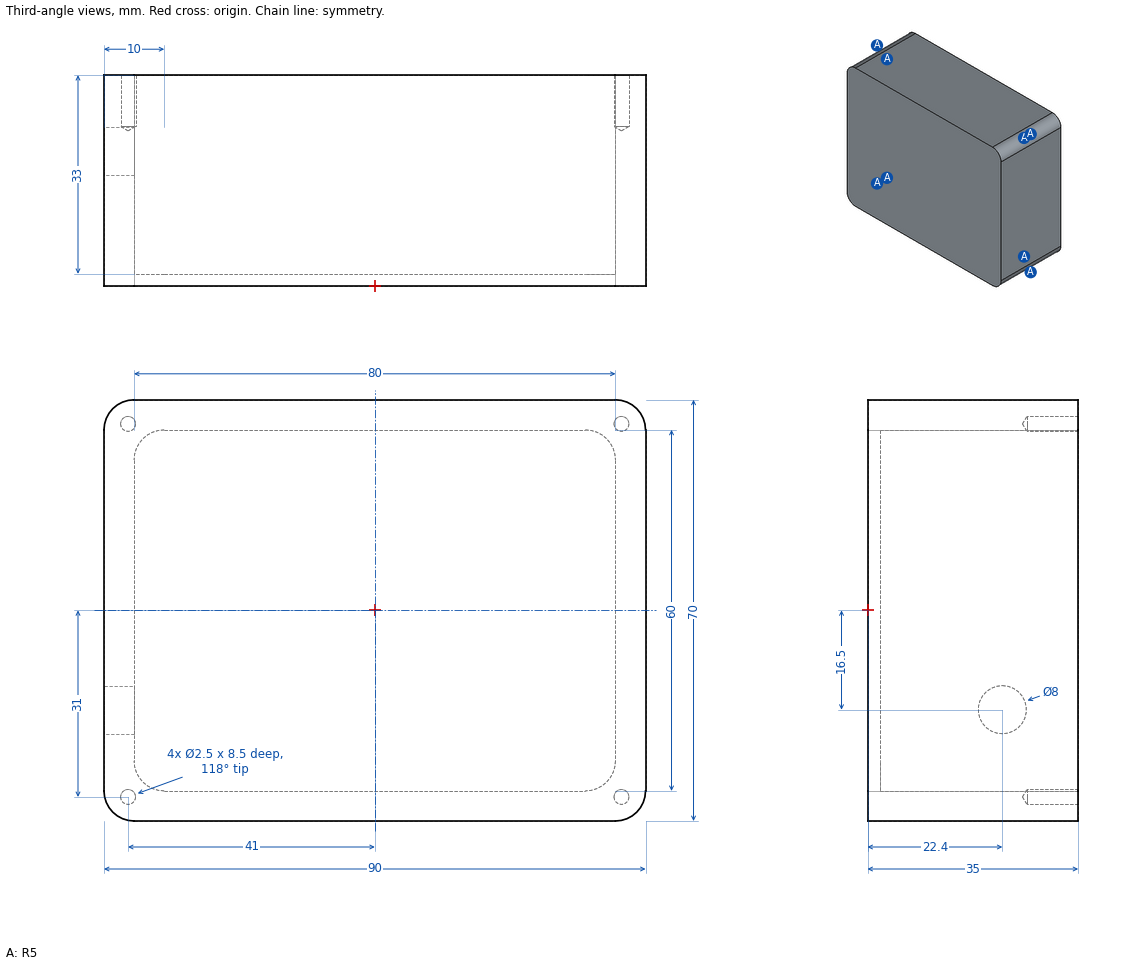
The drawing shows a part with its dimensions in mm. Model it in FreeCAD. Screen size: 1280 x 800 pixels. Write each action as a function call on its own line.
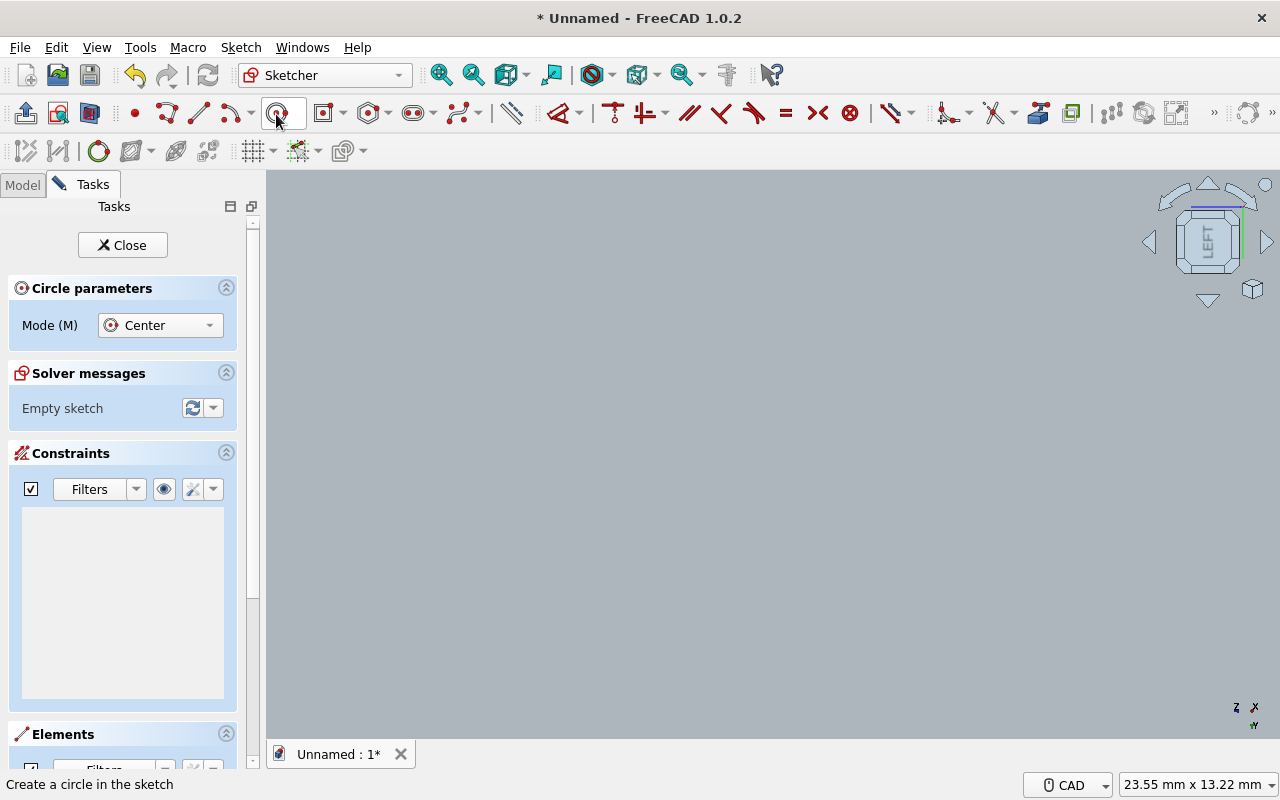
click(700, 448)
click(822, 327)
key(Escape)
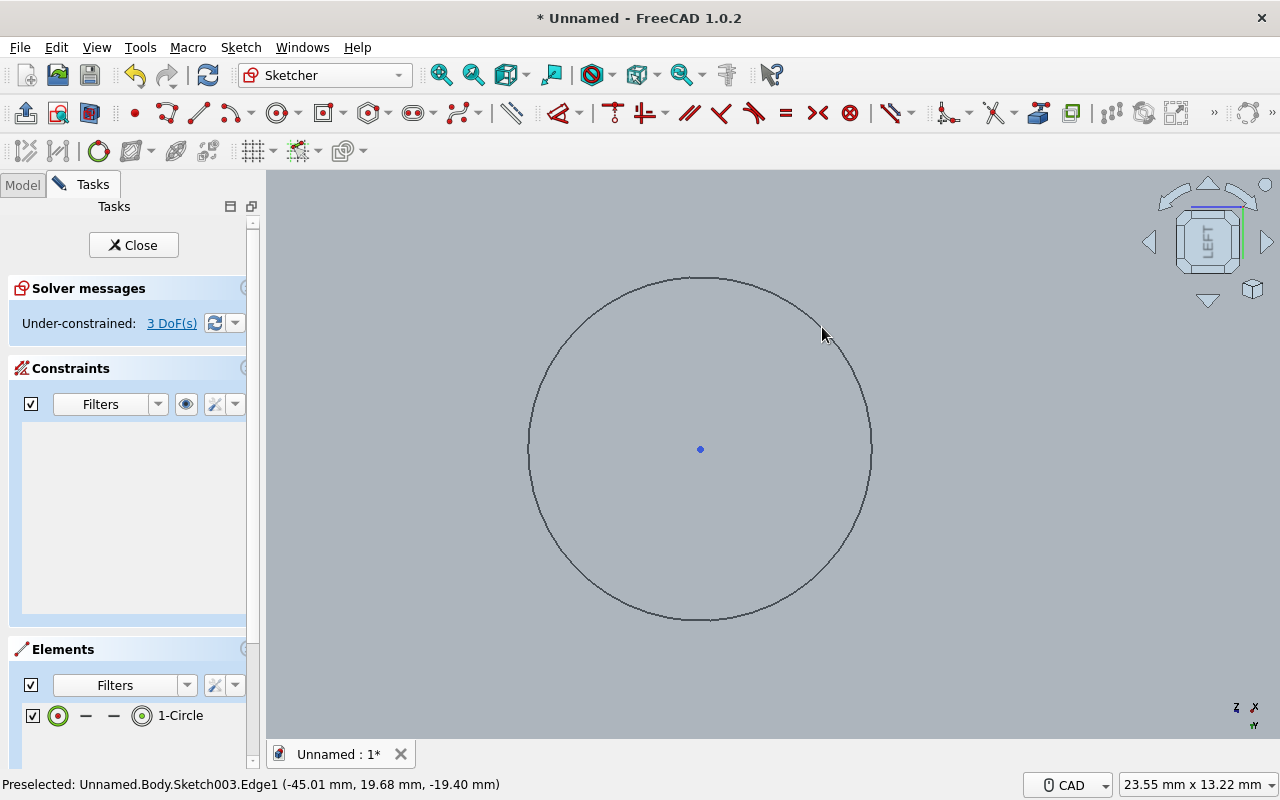
key(d)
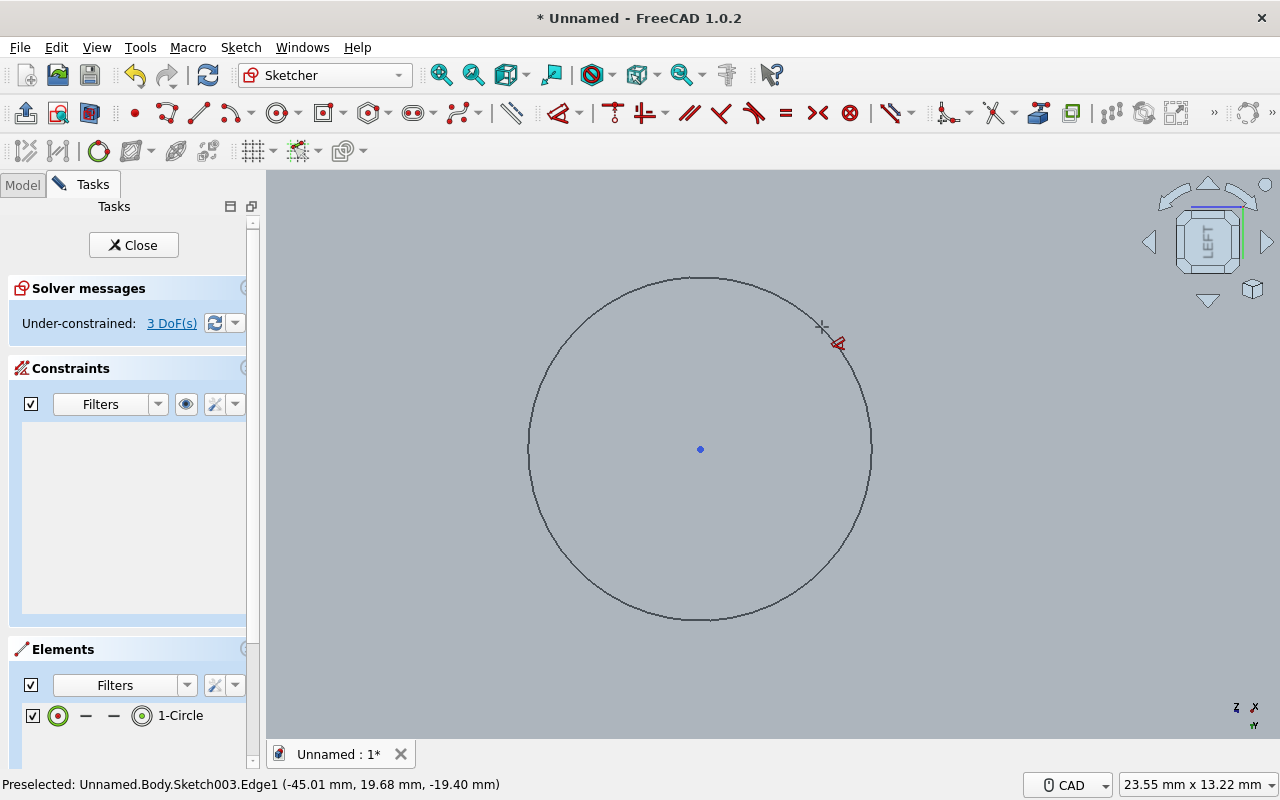
click(821, 327)
click(844, 304)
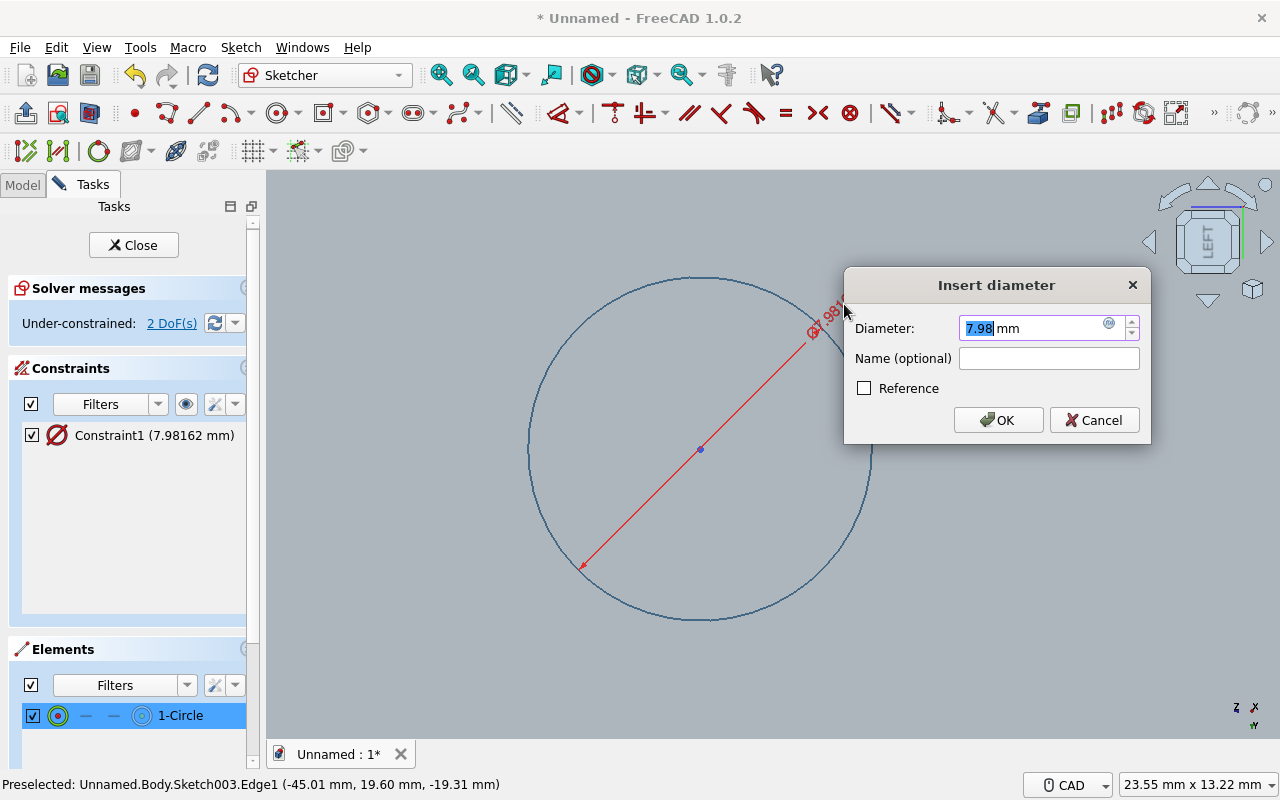
text(8)
key(Return)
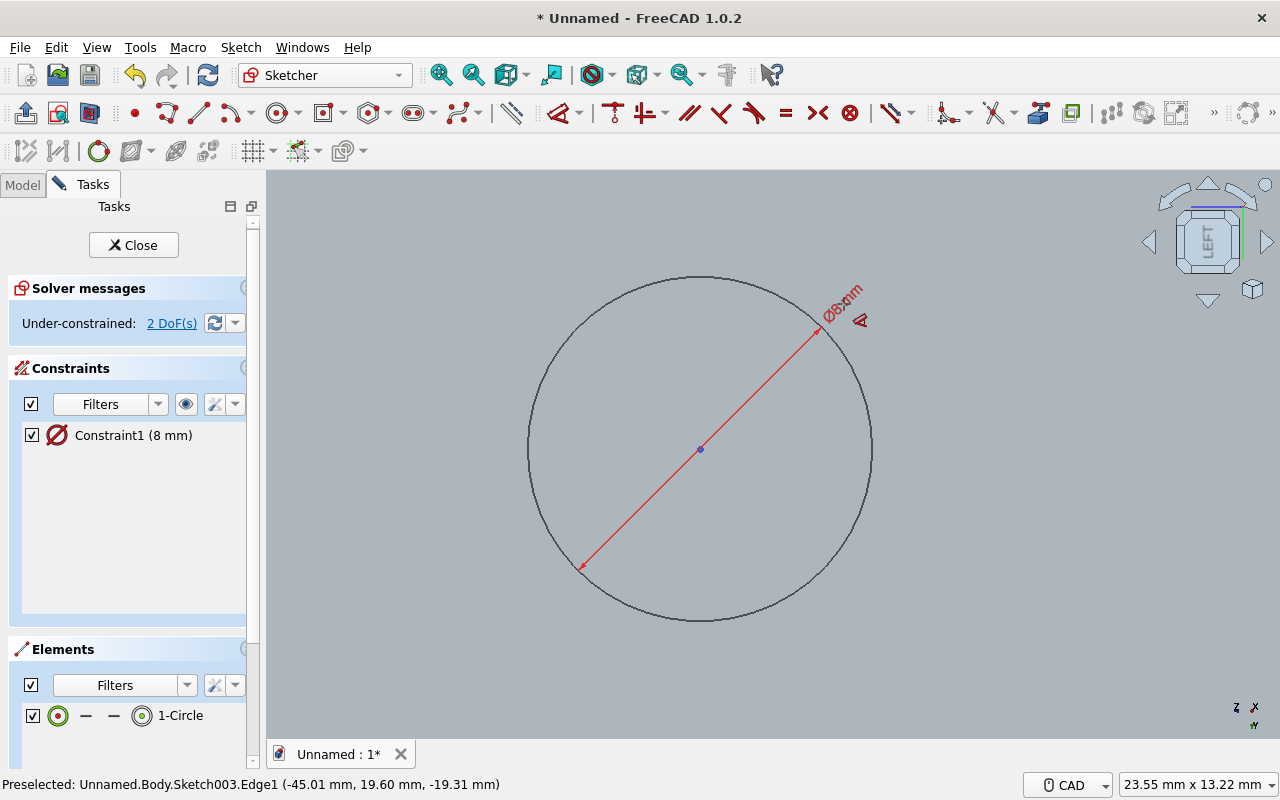
click(700, 449)
click(497, 483)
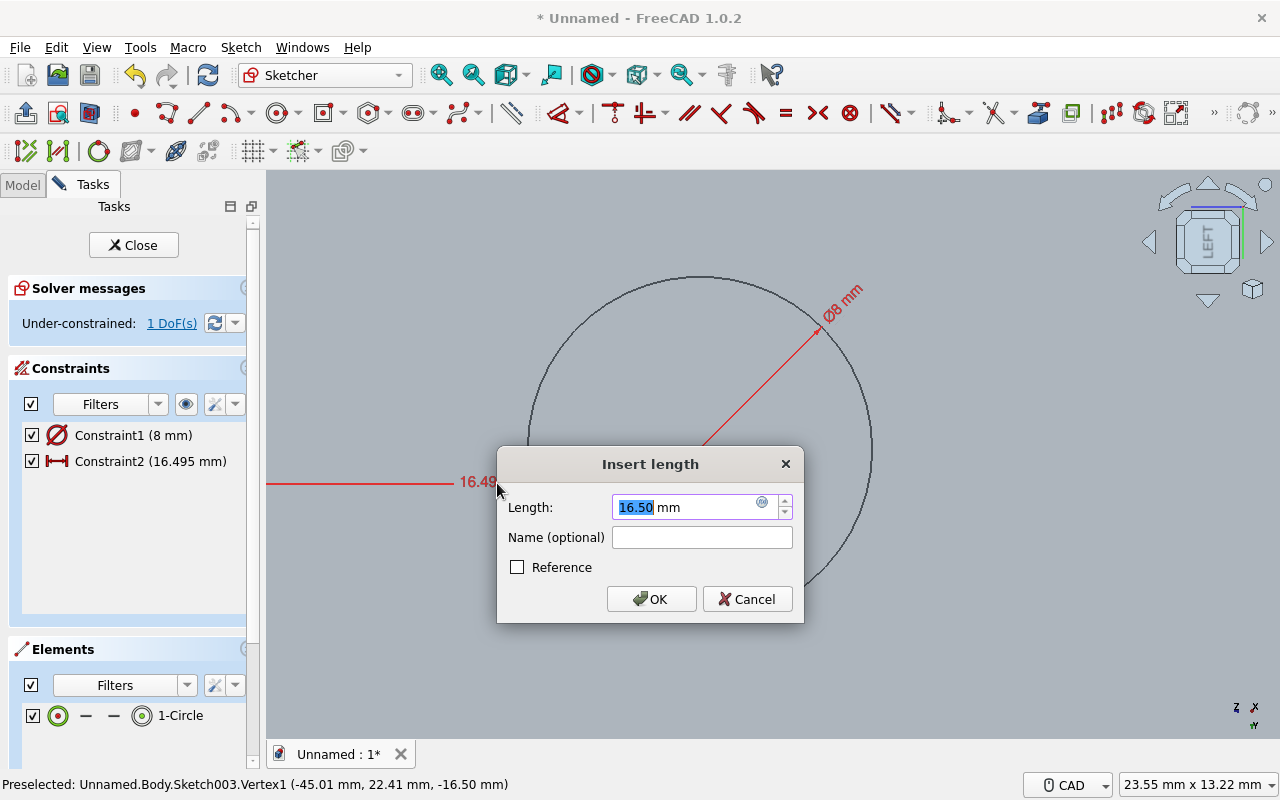
text(16.5)
key(Return)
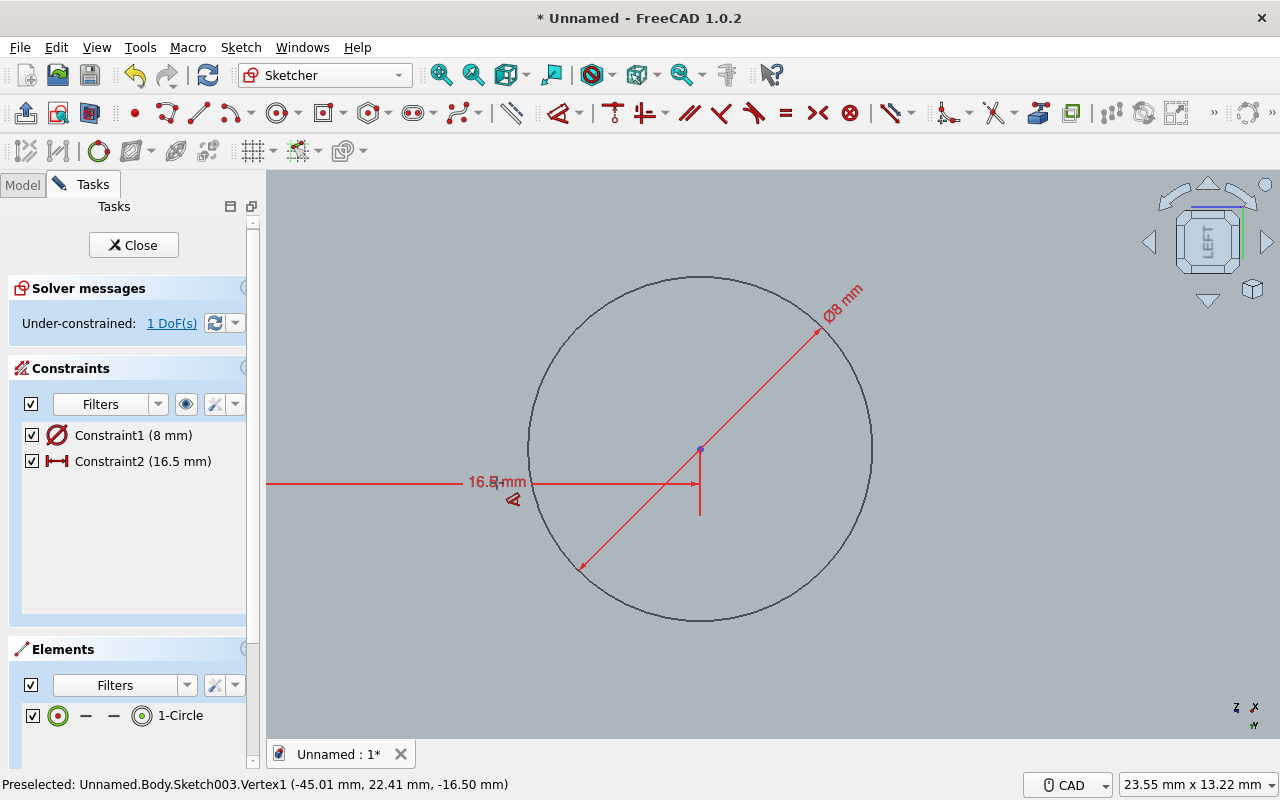
click(700, 449)
click(734, 323)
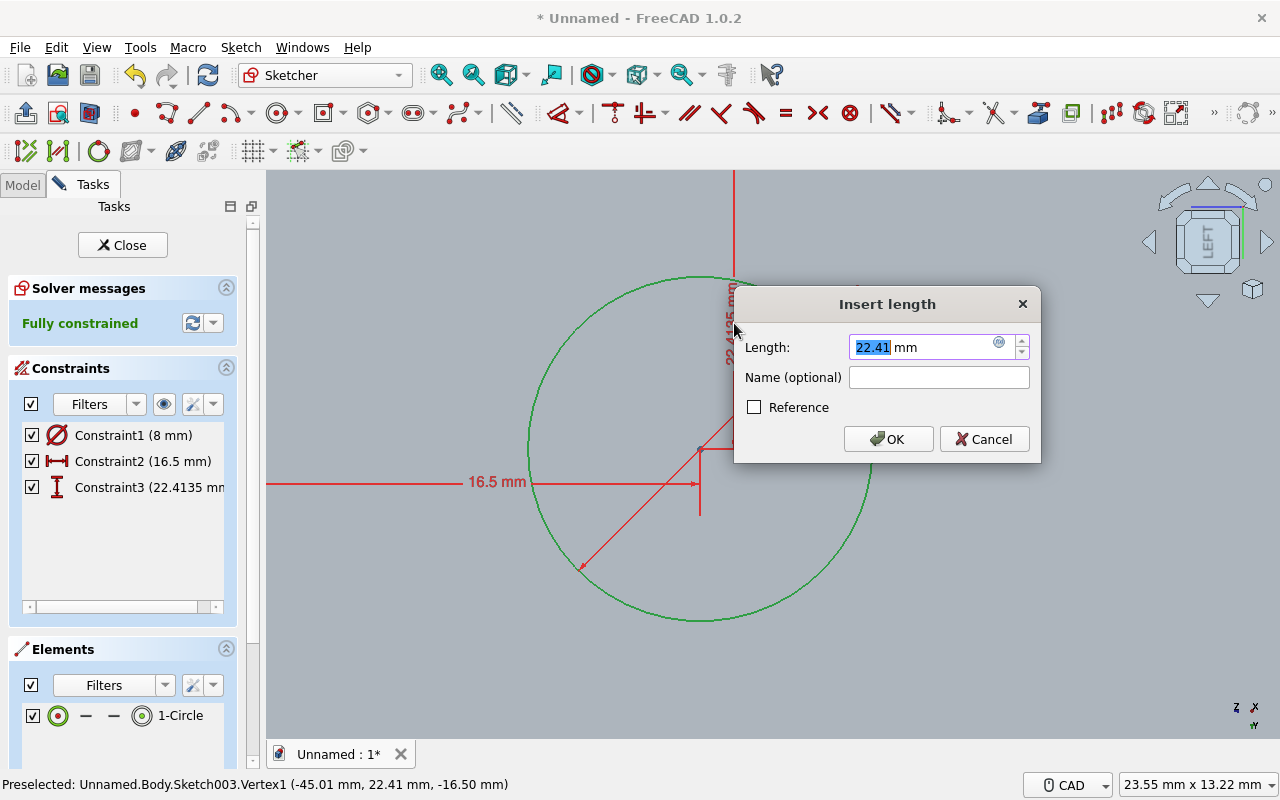
text(22.4)
key(Return)
key(Escape)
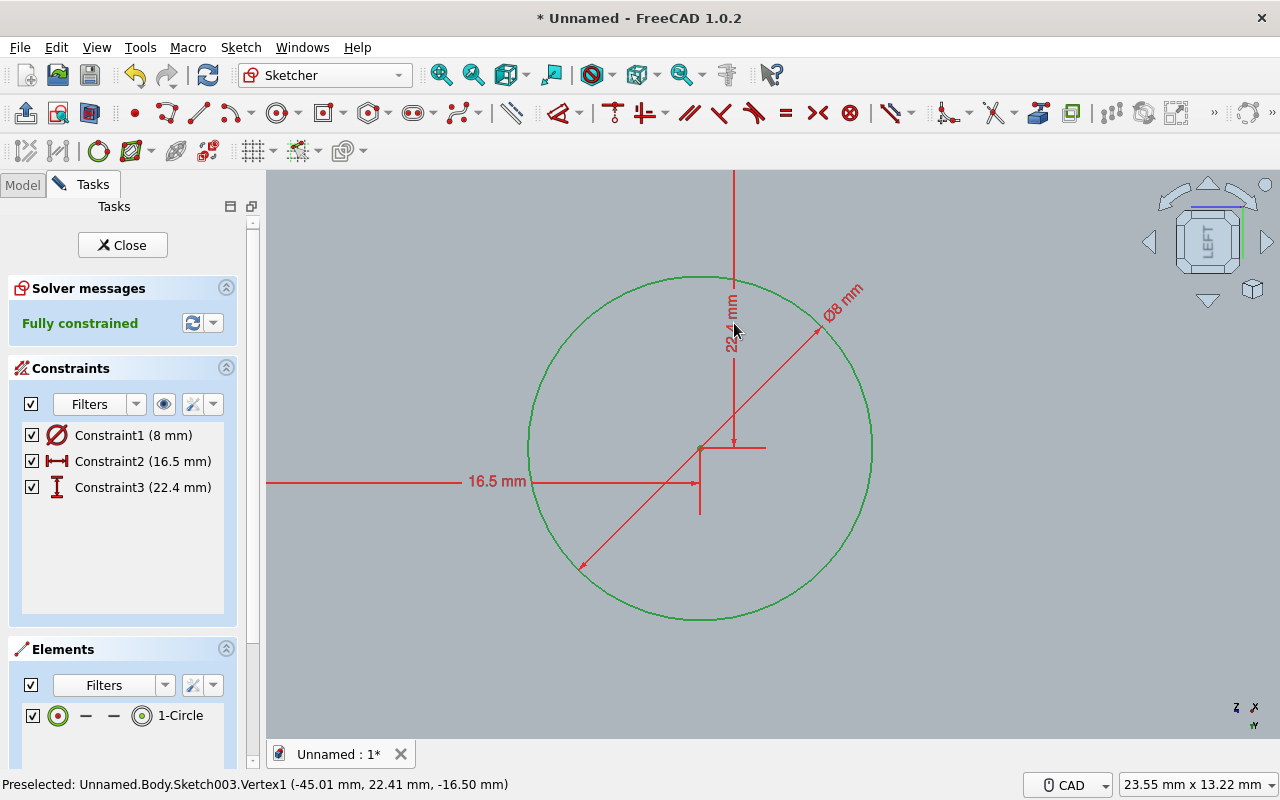
click(123, 245)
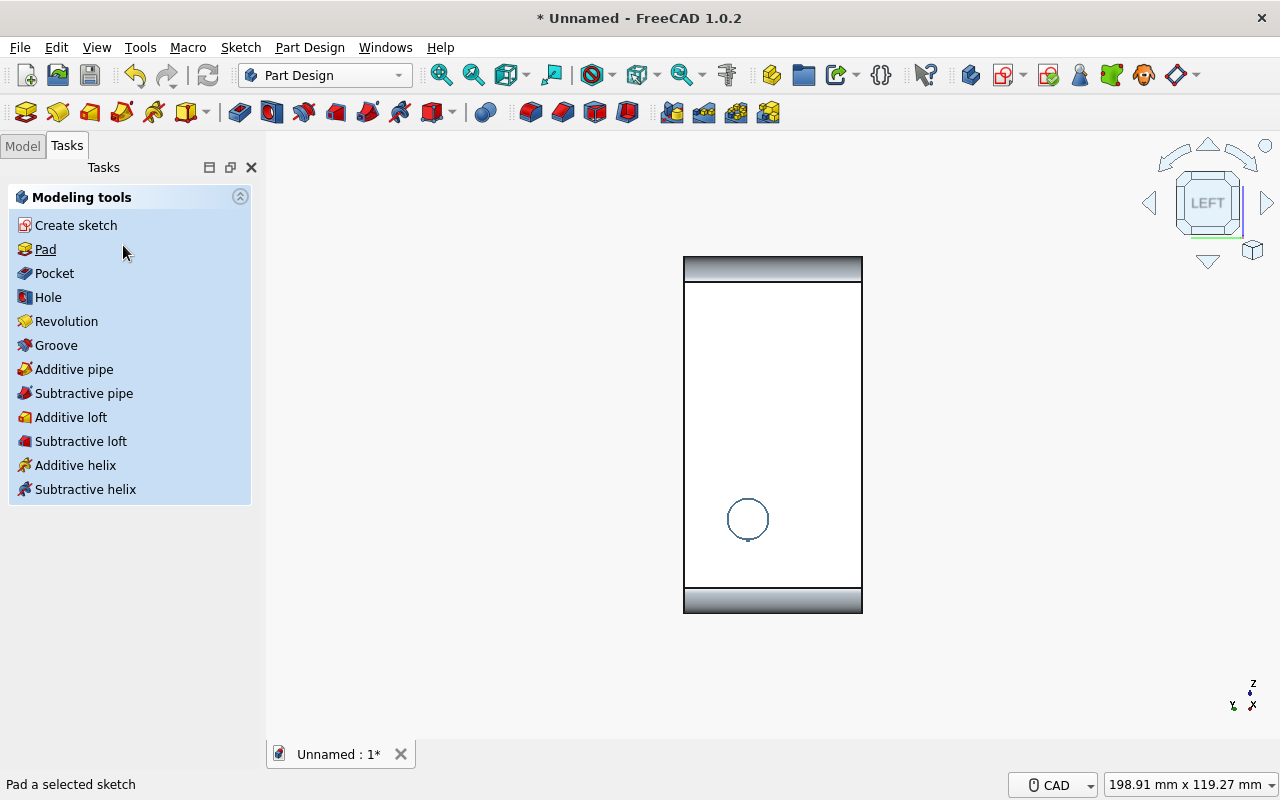
click(240, 112)